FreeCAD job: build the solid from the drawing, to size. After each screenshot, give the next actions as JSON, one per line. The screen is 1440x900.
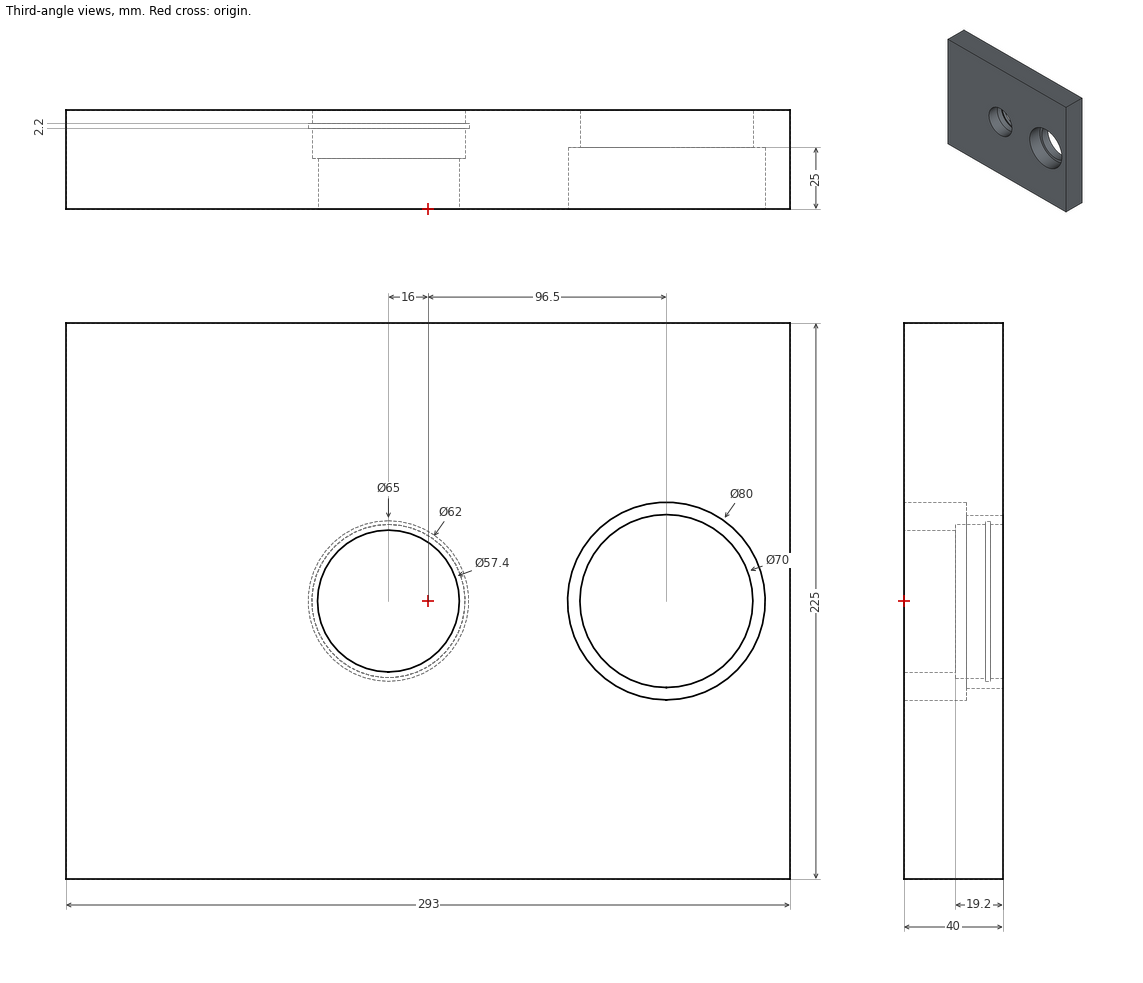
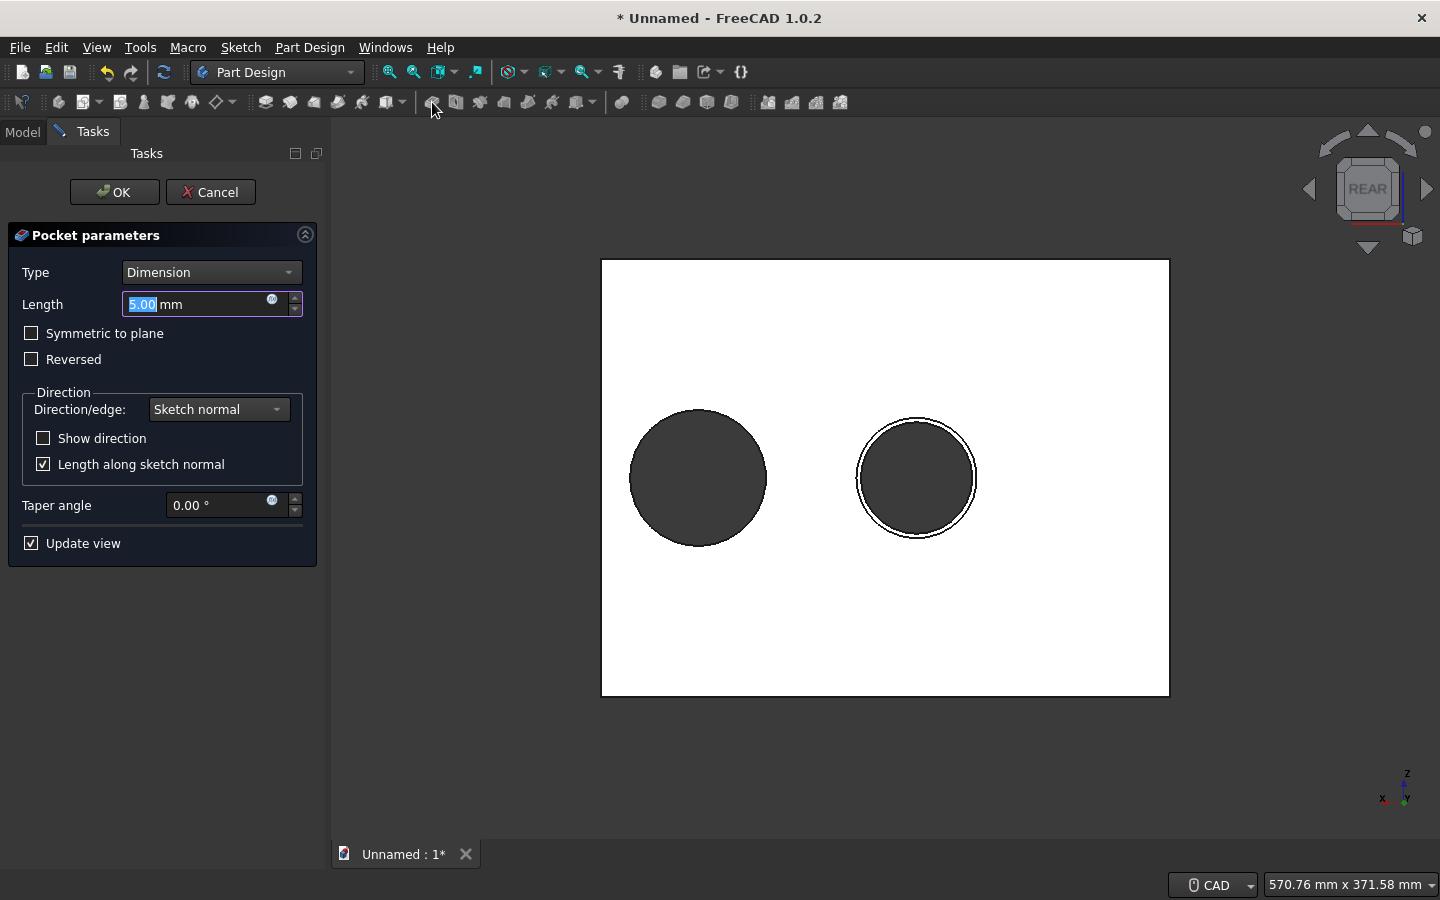
{"action": "type", "text": "19.2"}
{"action": "key", "text": "Tab"}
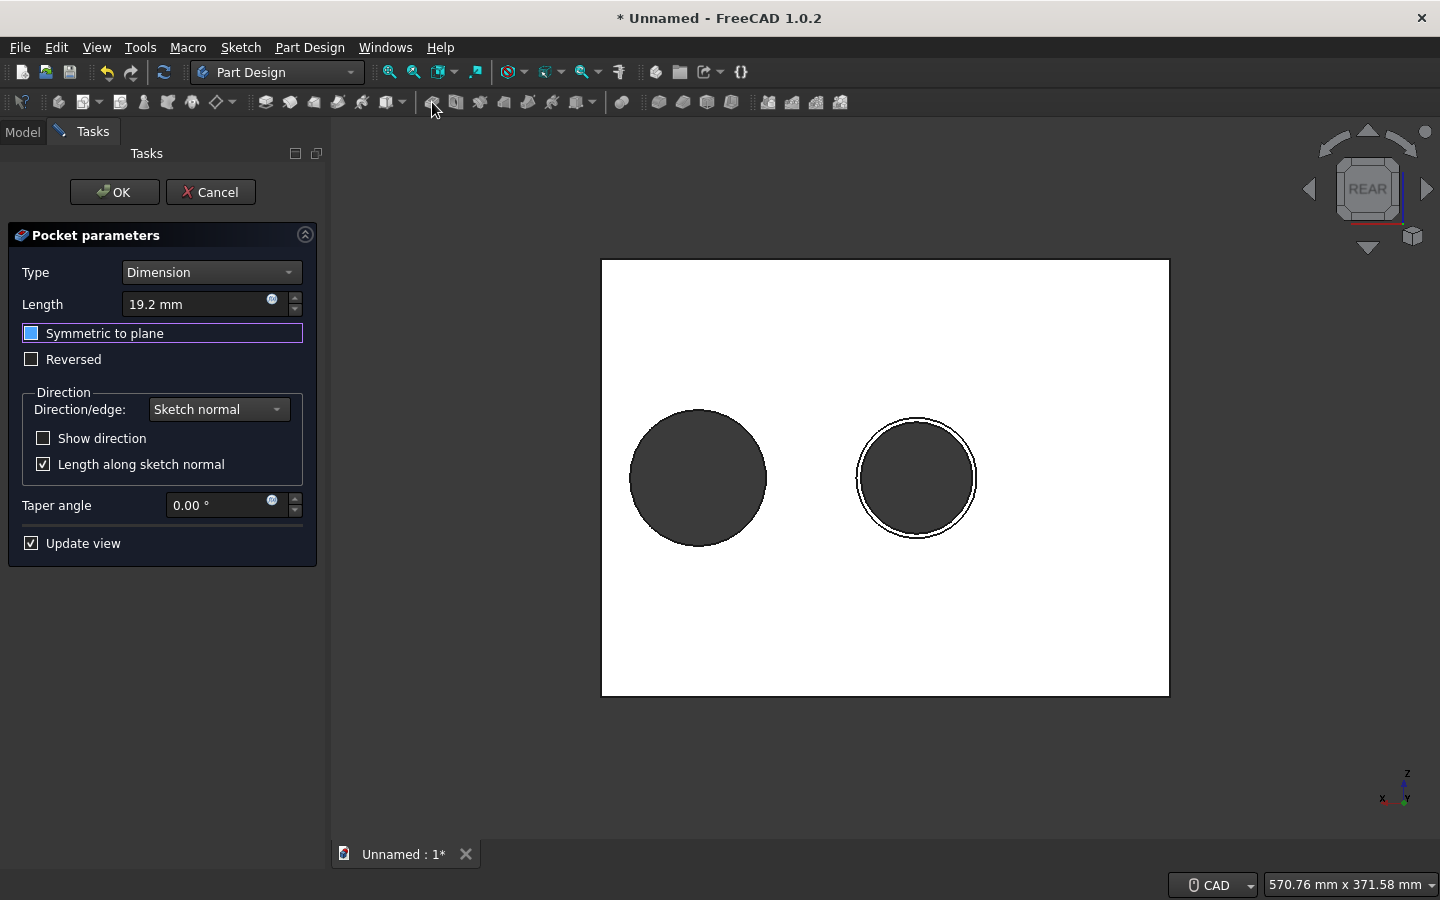
{"action": "left_click", "coordinate": [115, 192]}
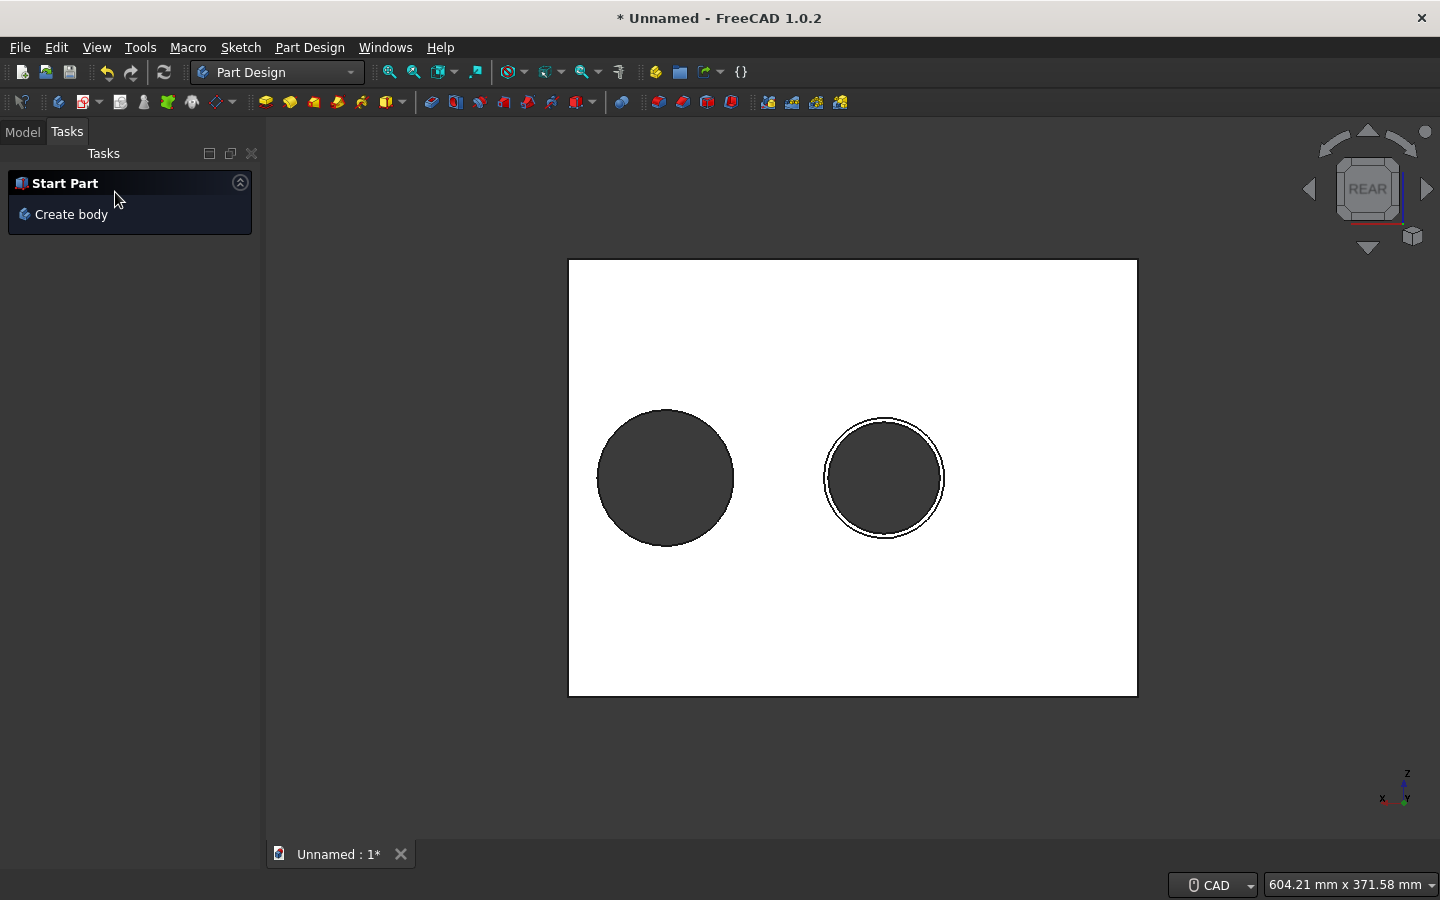
{"action": "left_click", "coordinate": [23, 131]}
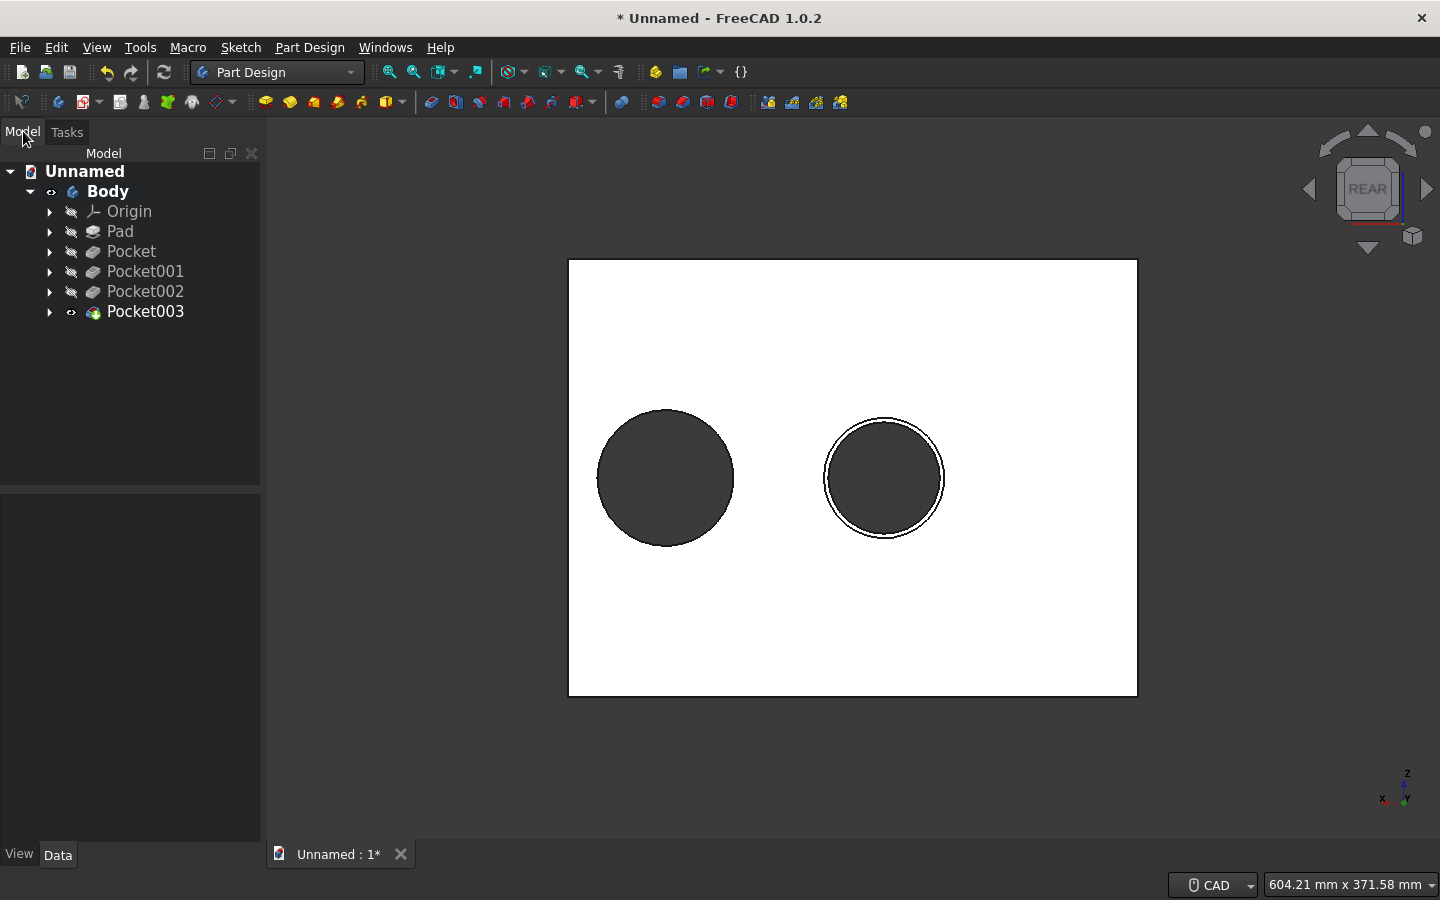
{"action": "left_click", "coordinate": [50, 212]}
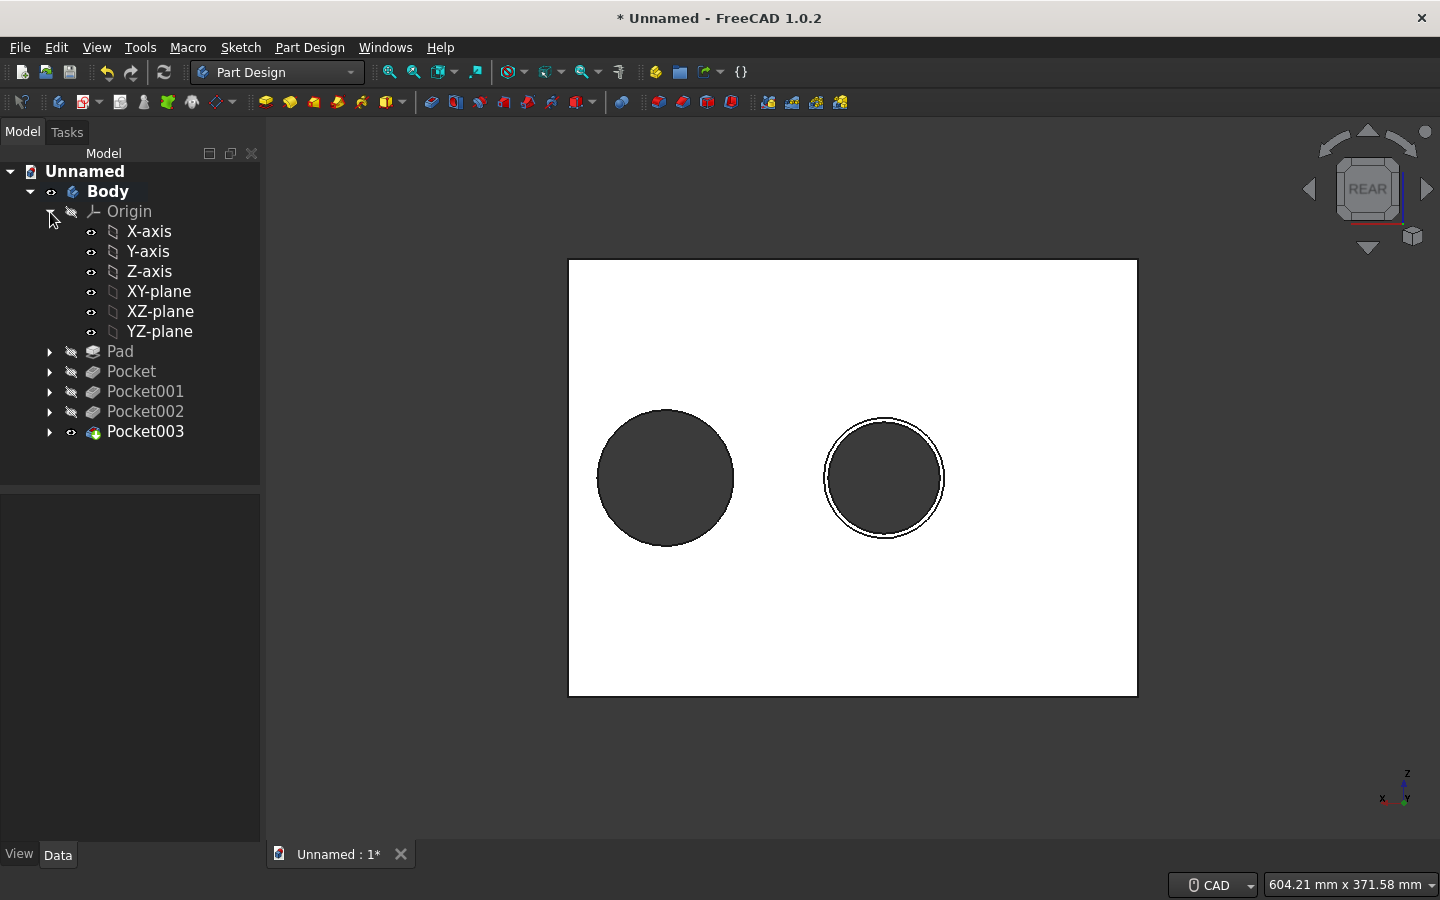
{"action": "left_click", "coordinate": [136, 312]}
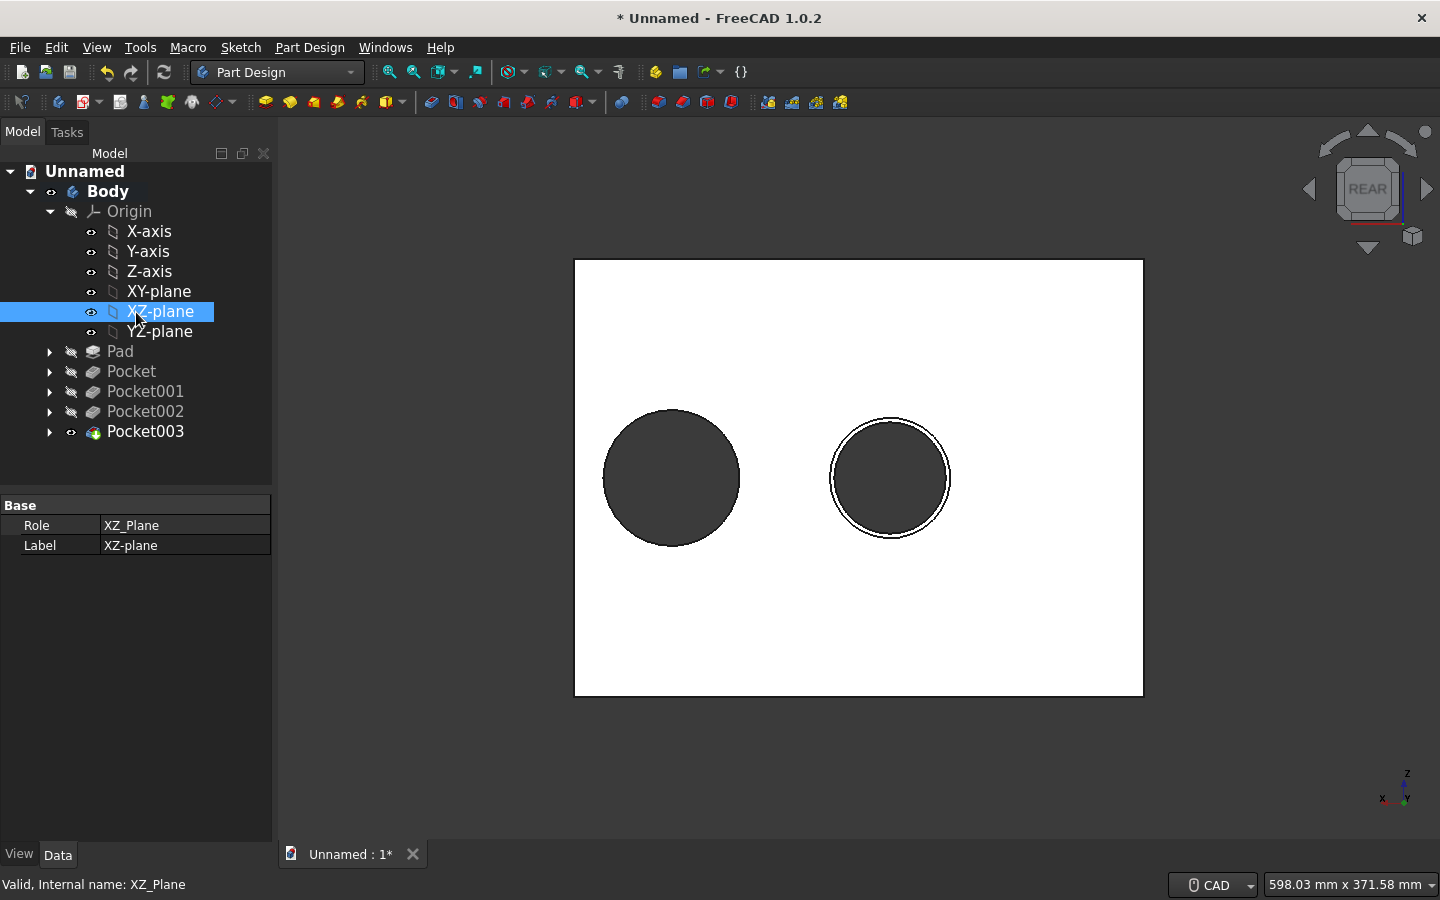
{"action": "left_click", "coordinate": [216, 102]}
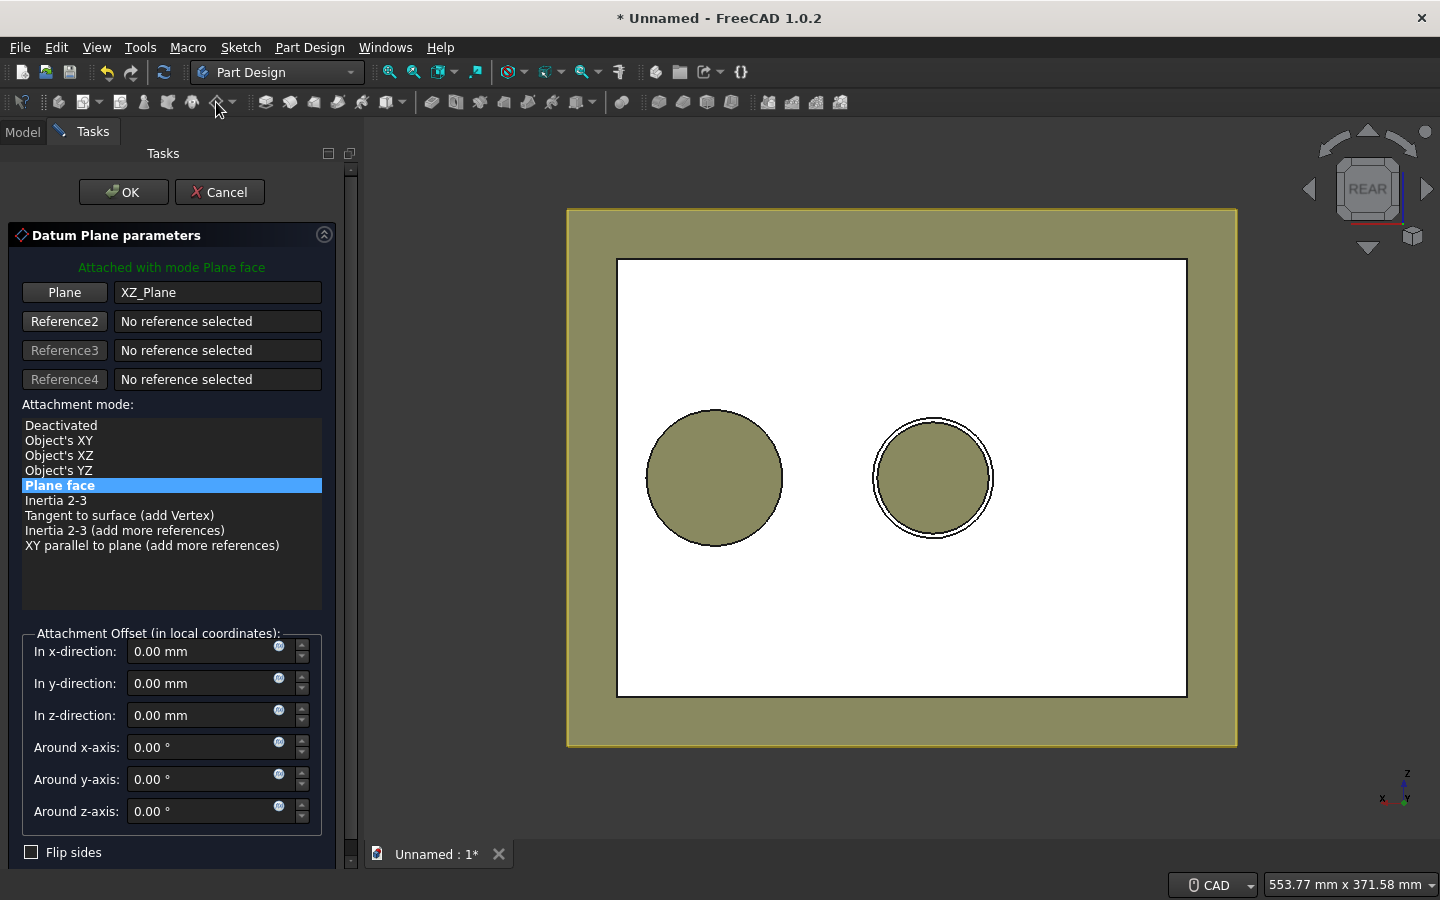
{"action": "triple_click", "coordinate": [210, 715]}